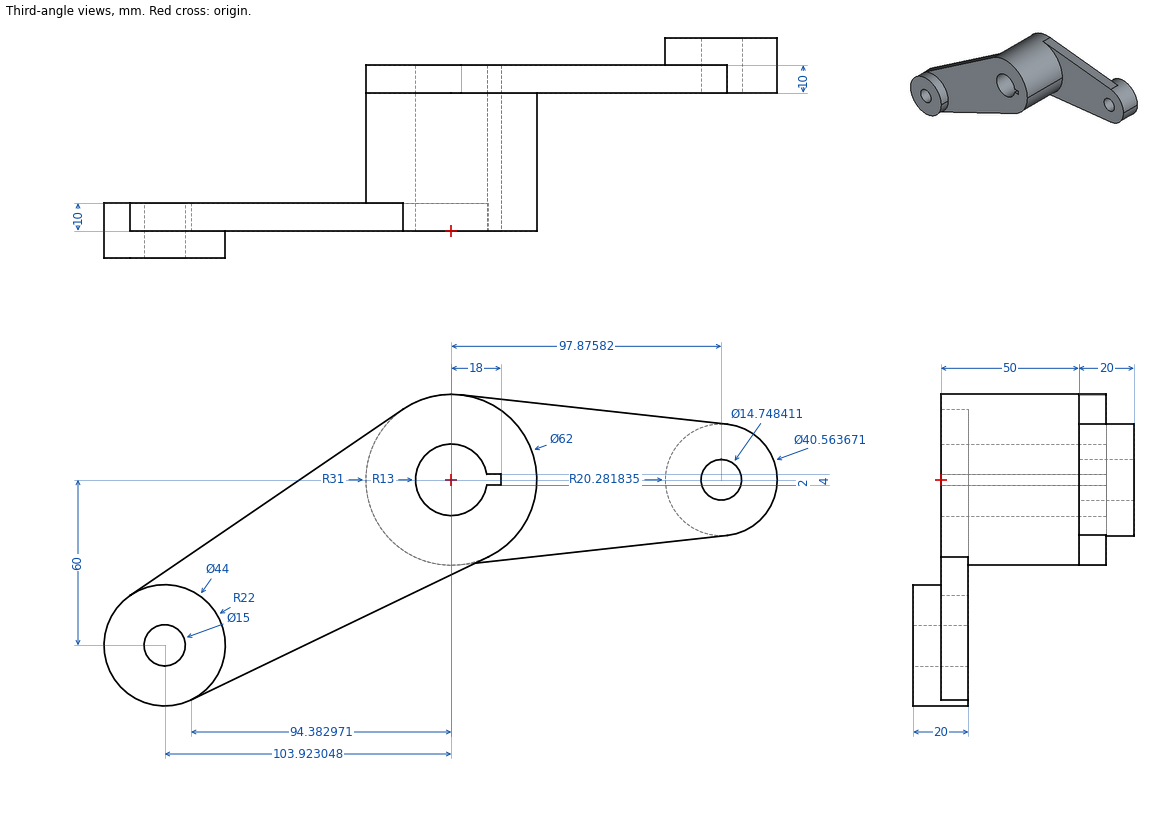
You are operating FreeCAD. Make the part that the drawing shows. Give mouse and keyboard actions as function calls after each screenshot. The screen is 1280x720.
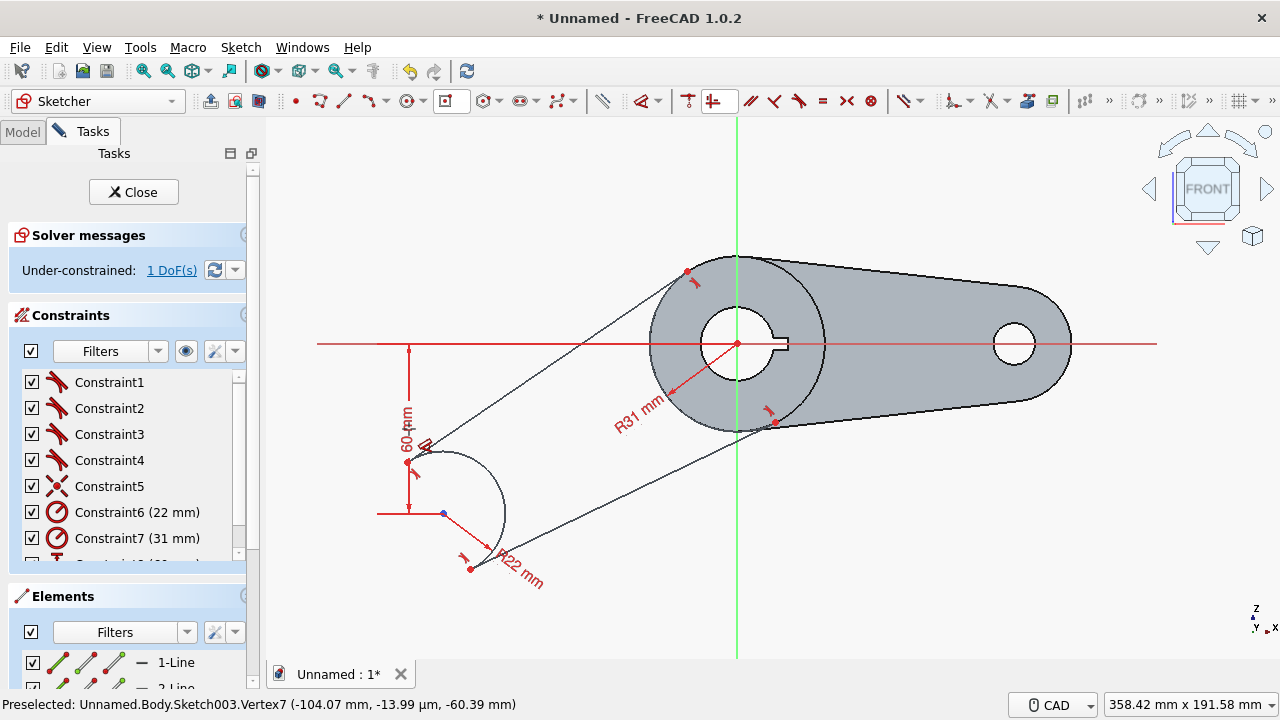
click(470, 570)
click(604, 604)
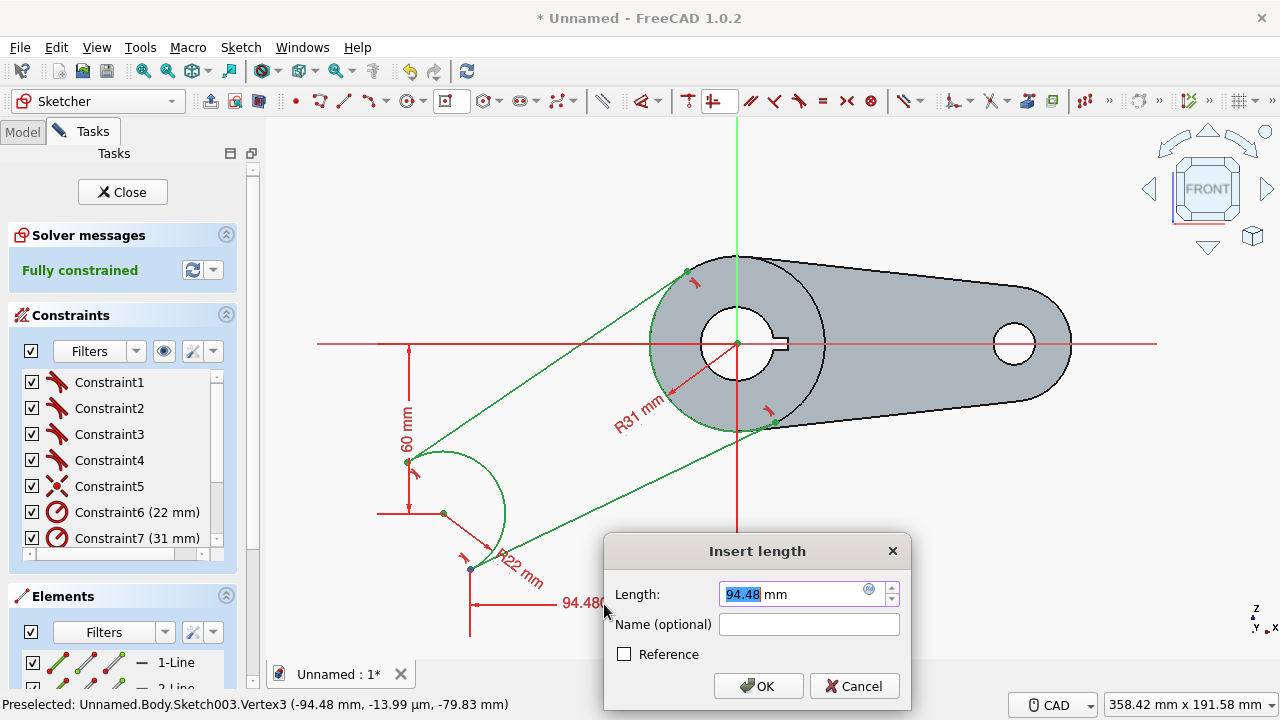
text(94.382971)
key(Return)
key(Escape)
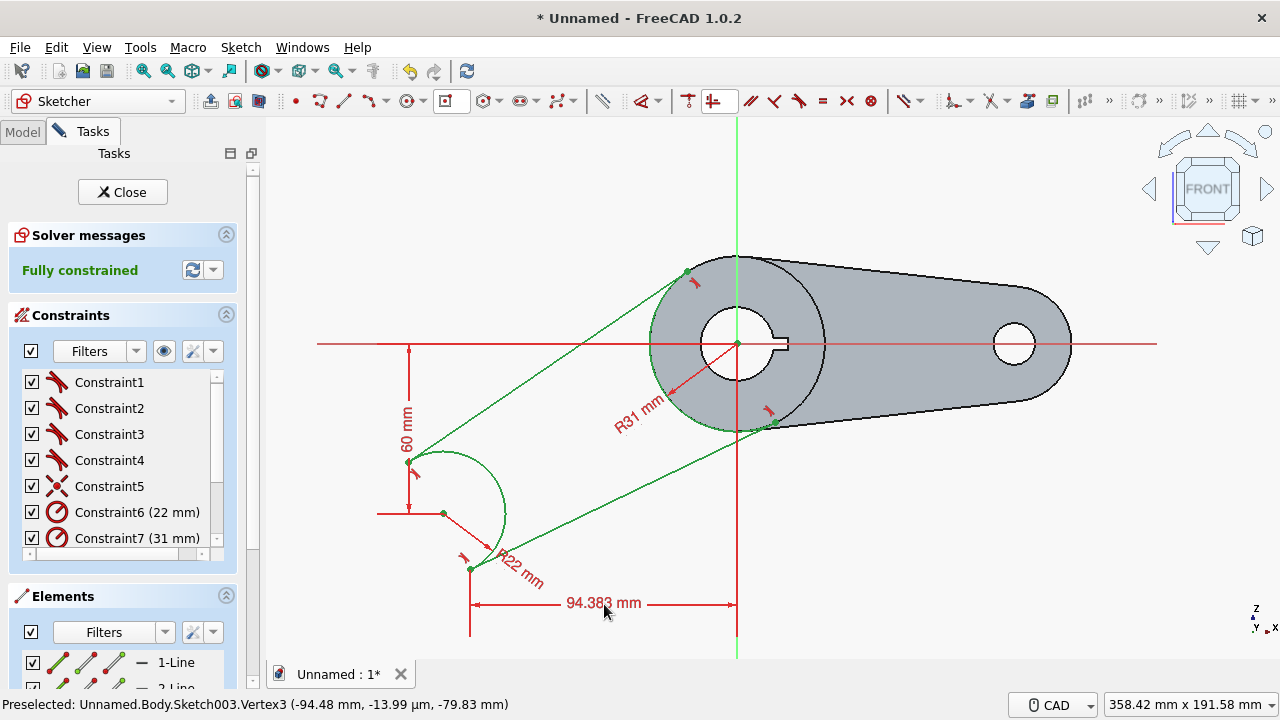
click(123, 192)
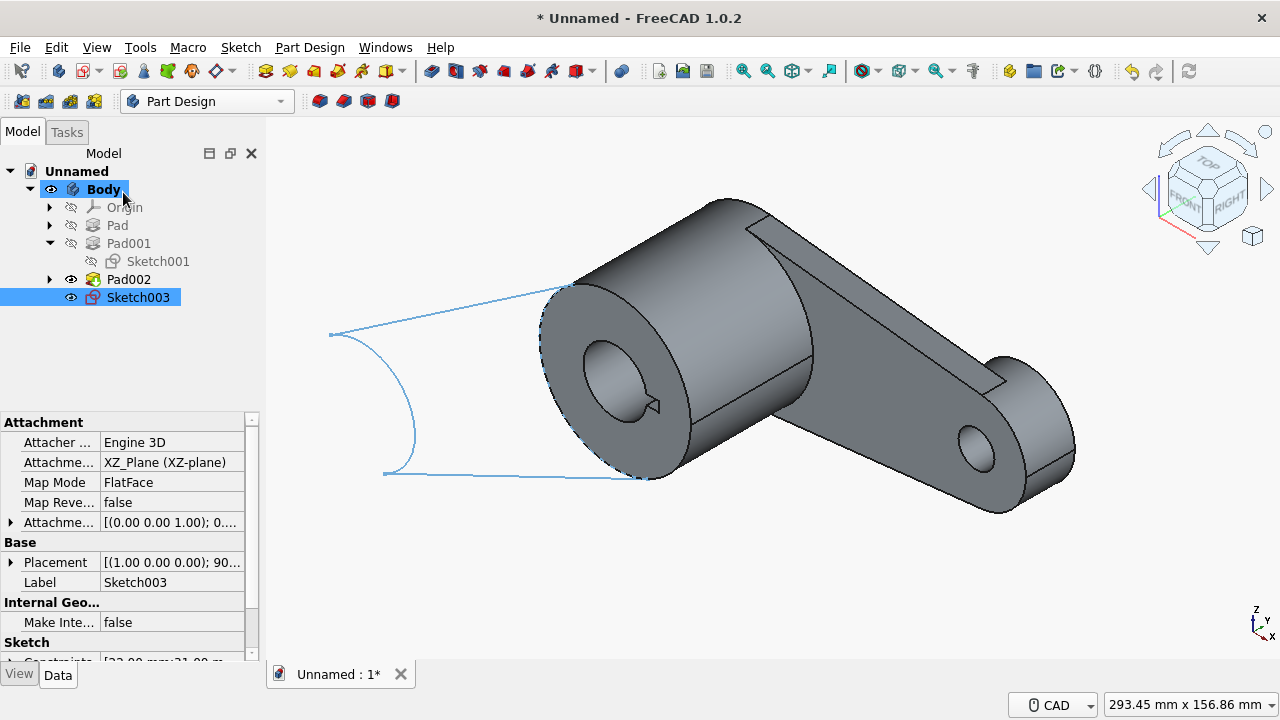
click(266, 72)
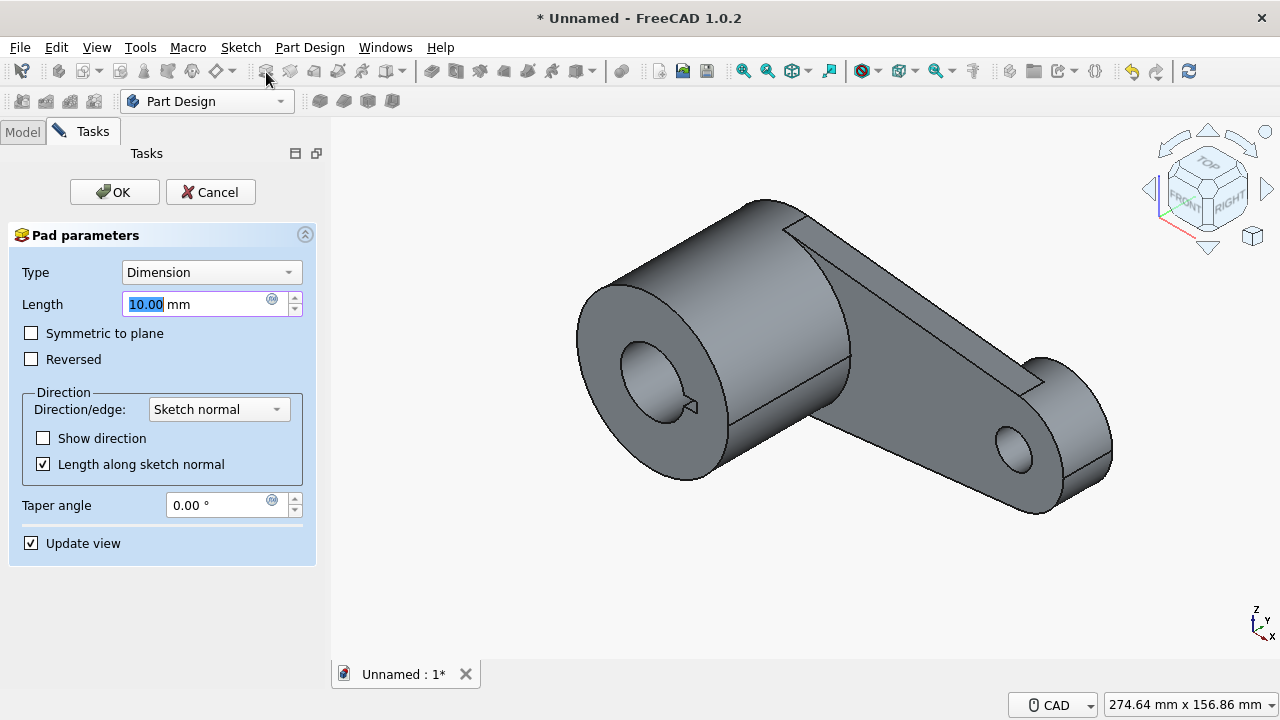
text(10)
key(Tab)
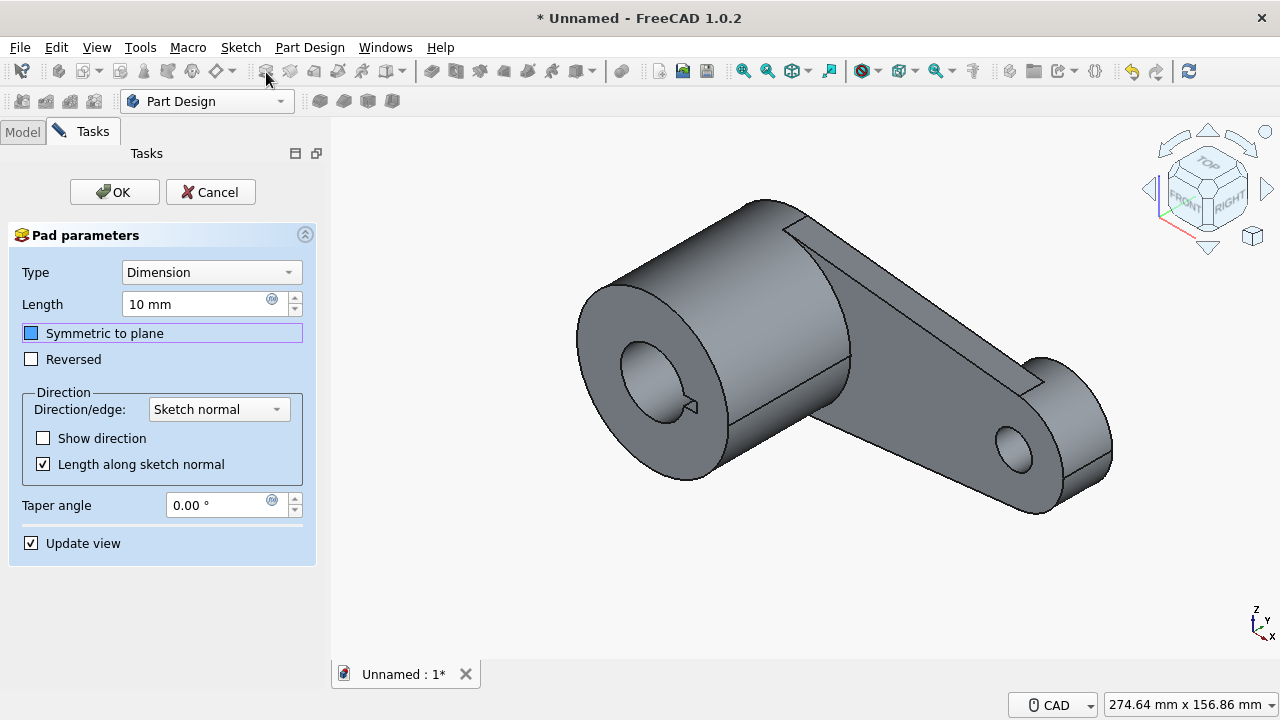
click(30, 359)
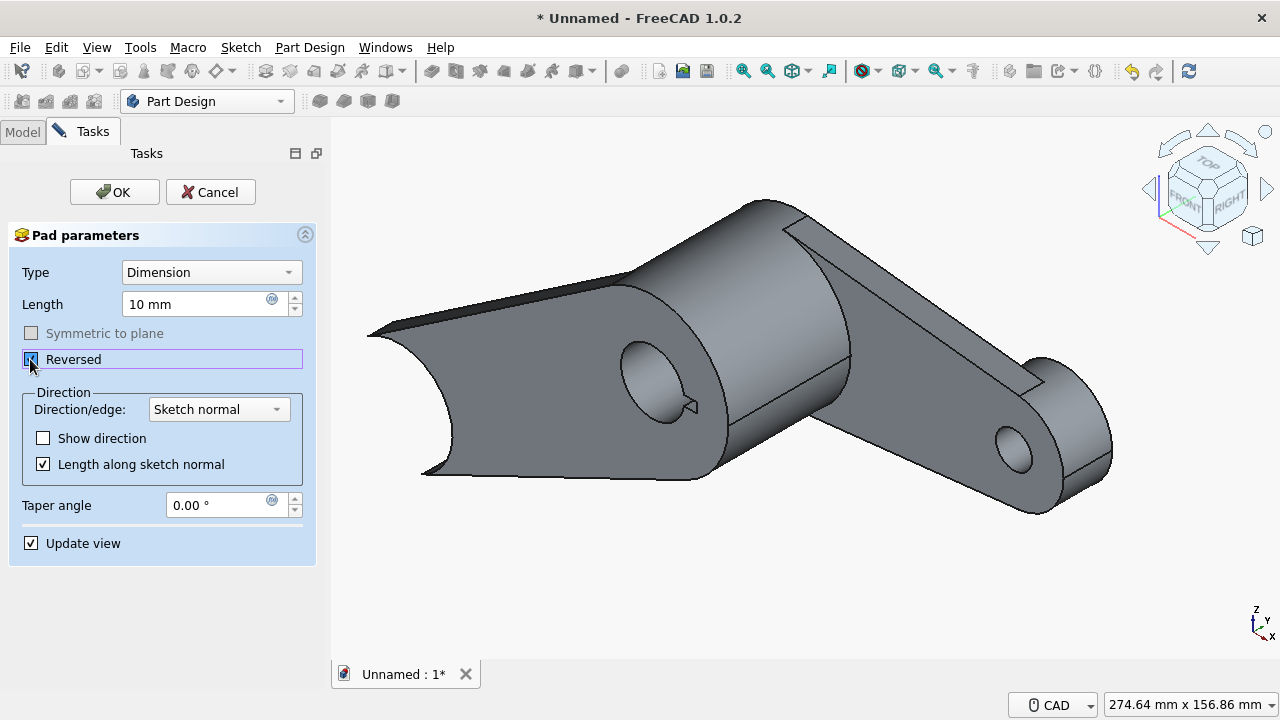
click(115, 192)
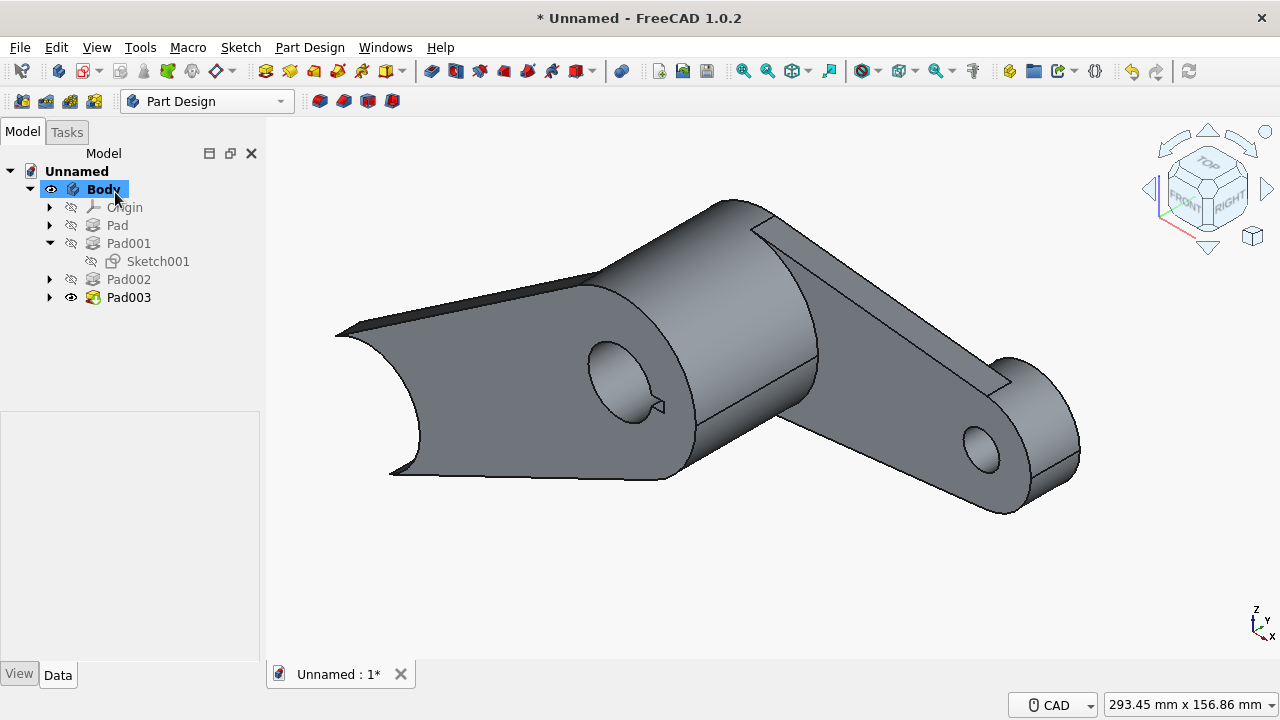
click(744, 72)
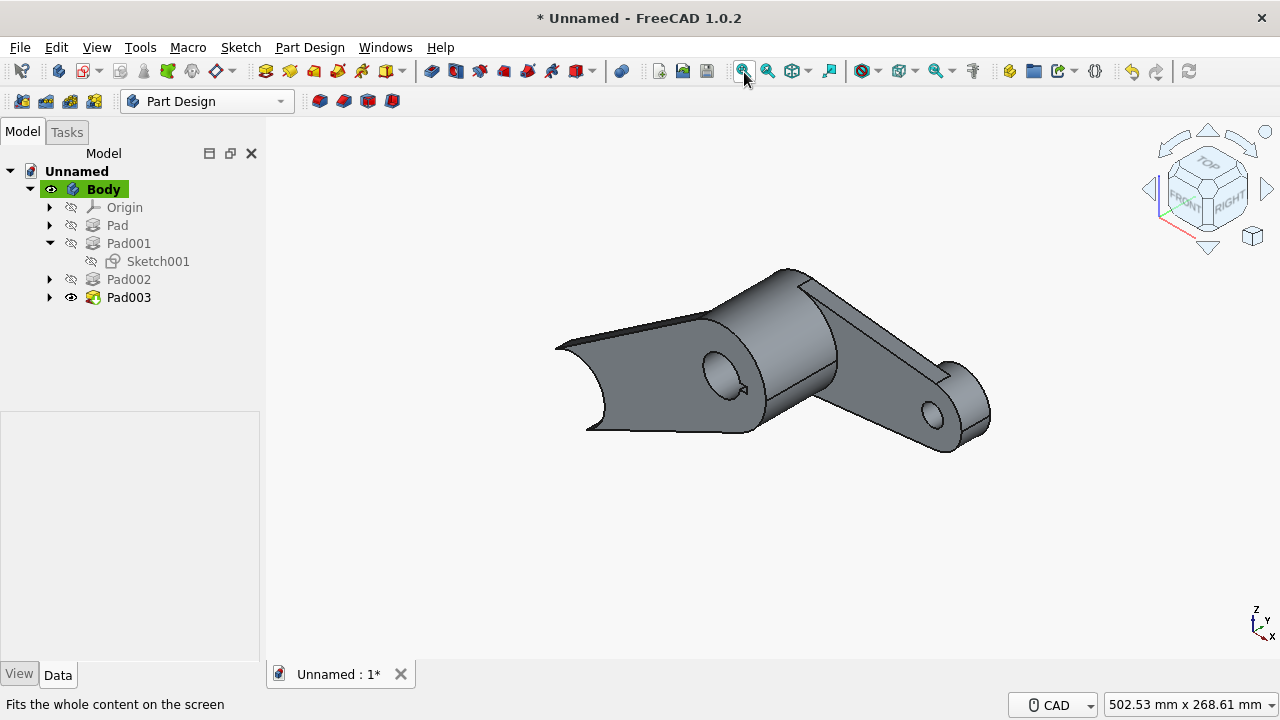
click(661, 380)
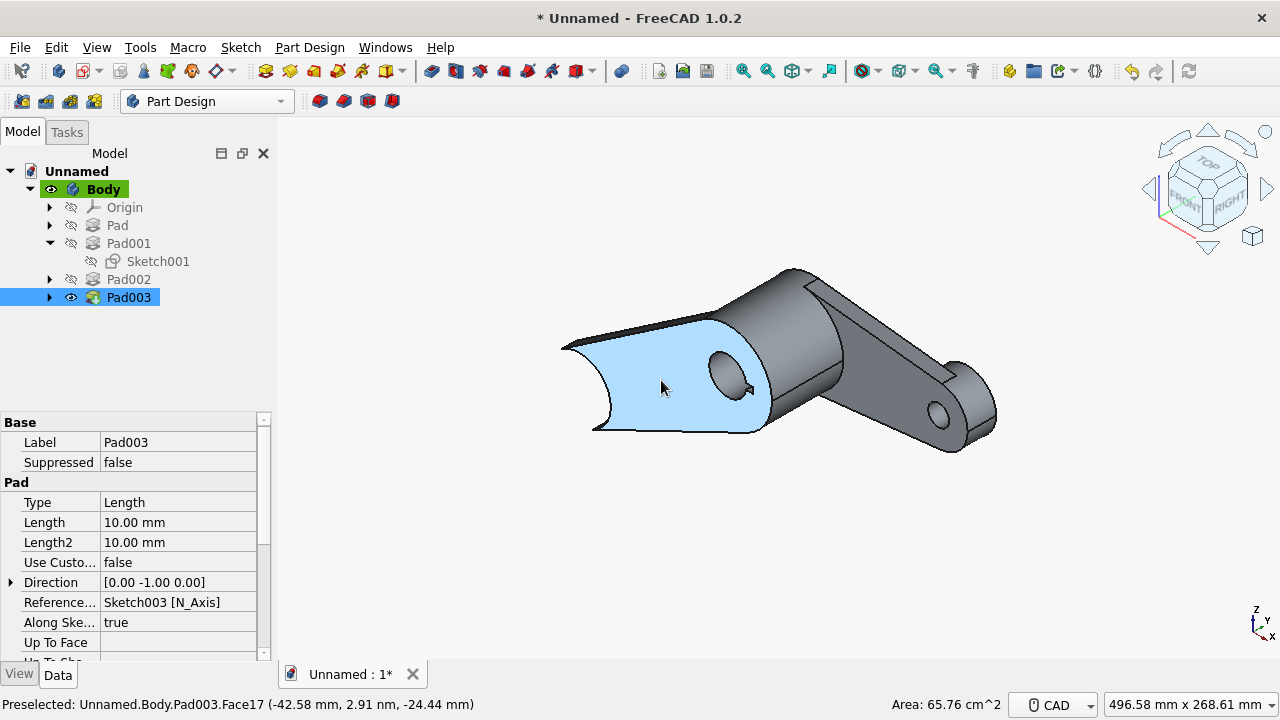
click(84, 72)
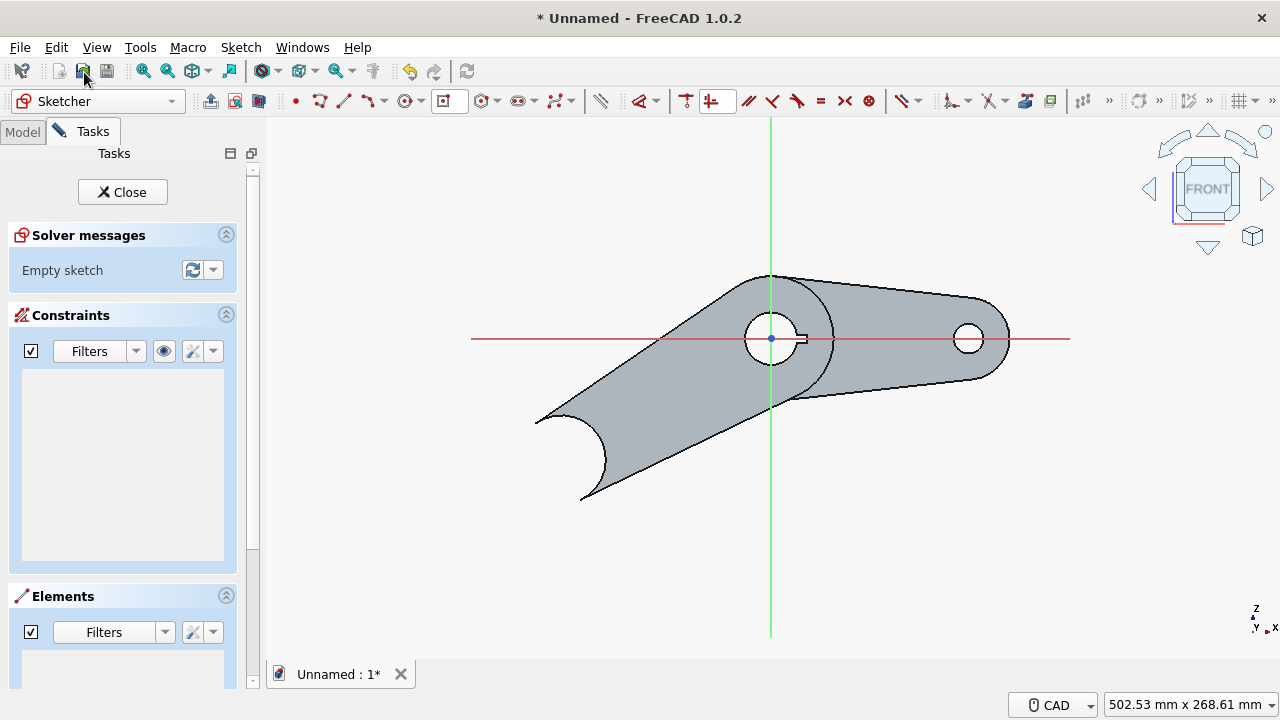
scroll(515, 483, up, 7)